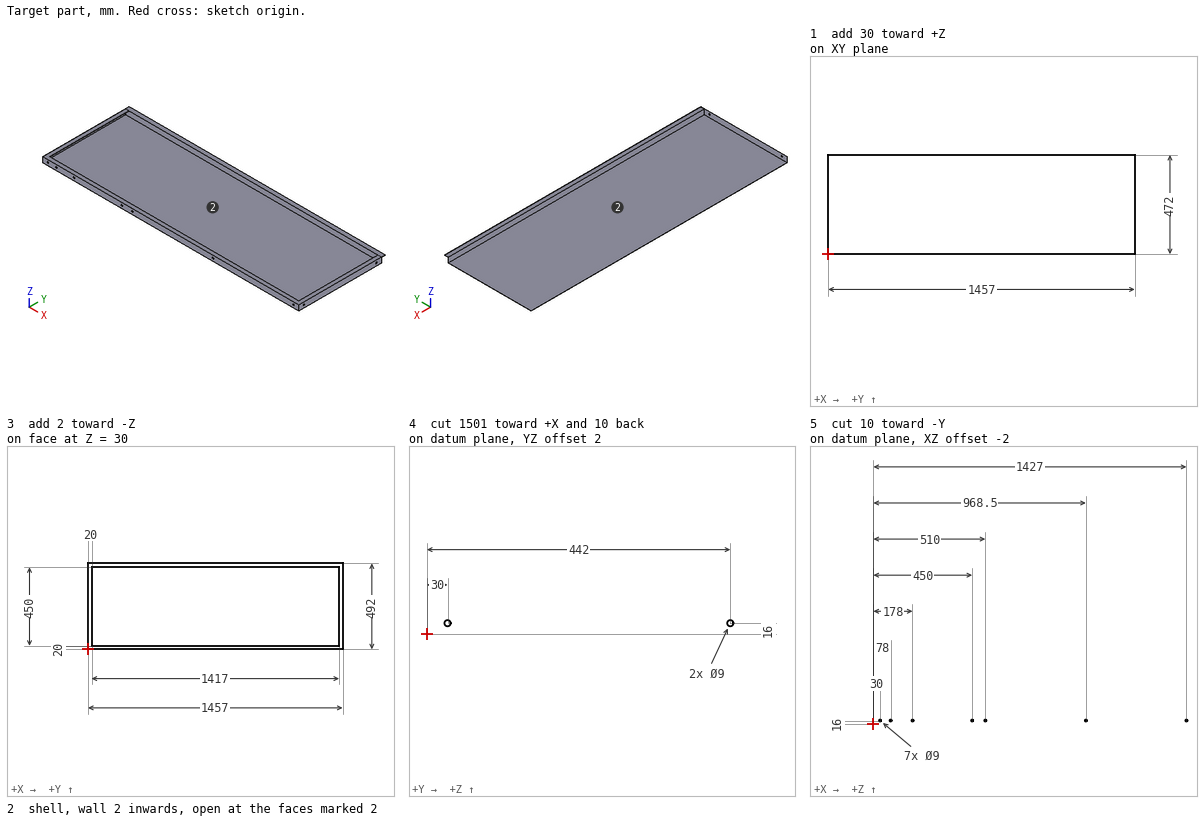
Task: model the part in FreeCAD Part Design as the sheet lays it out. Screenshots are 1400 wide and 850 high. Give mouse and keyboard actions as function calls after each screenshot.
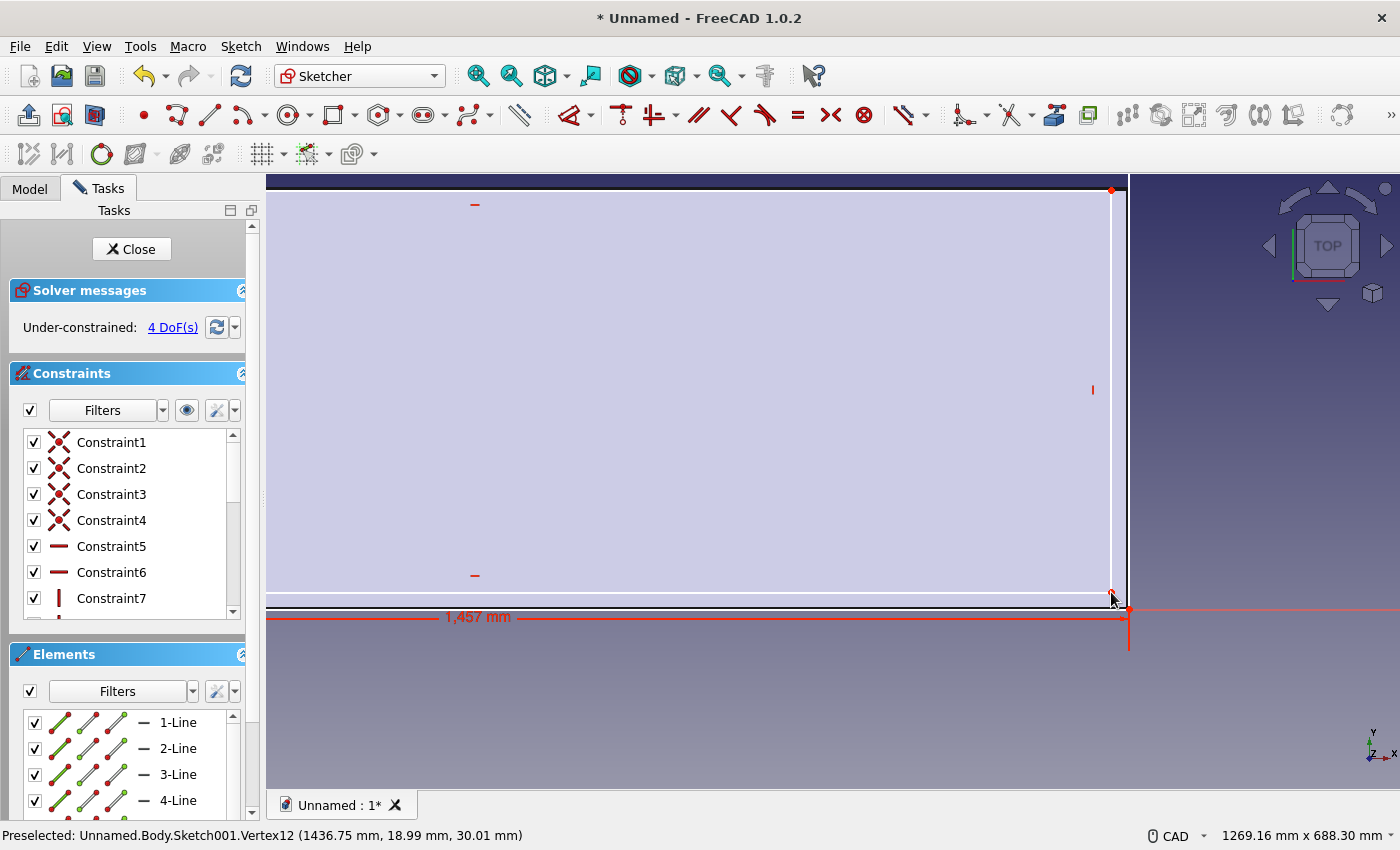
scroll(1113, 593, down, 3)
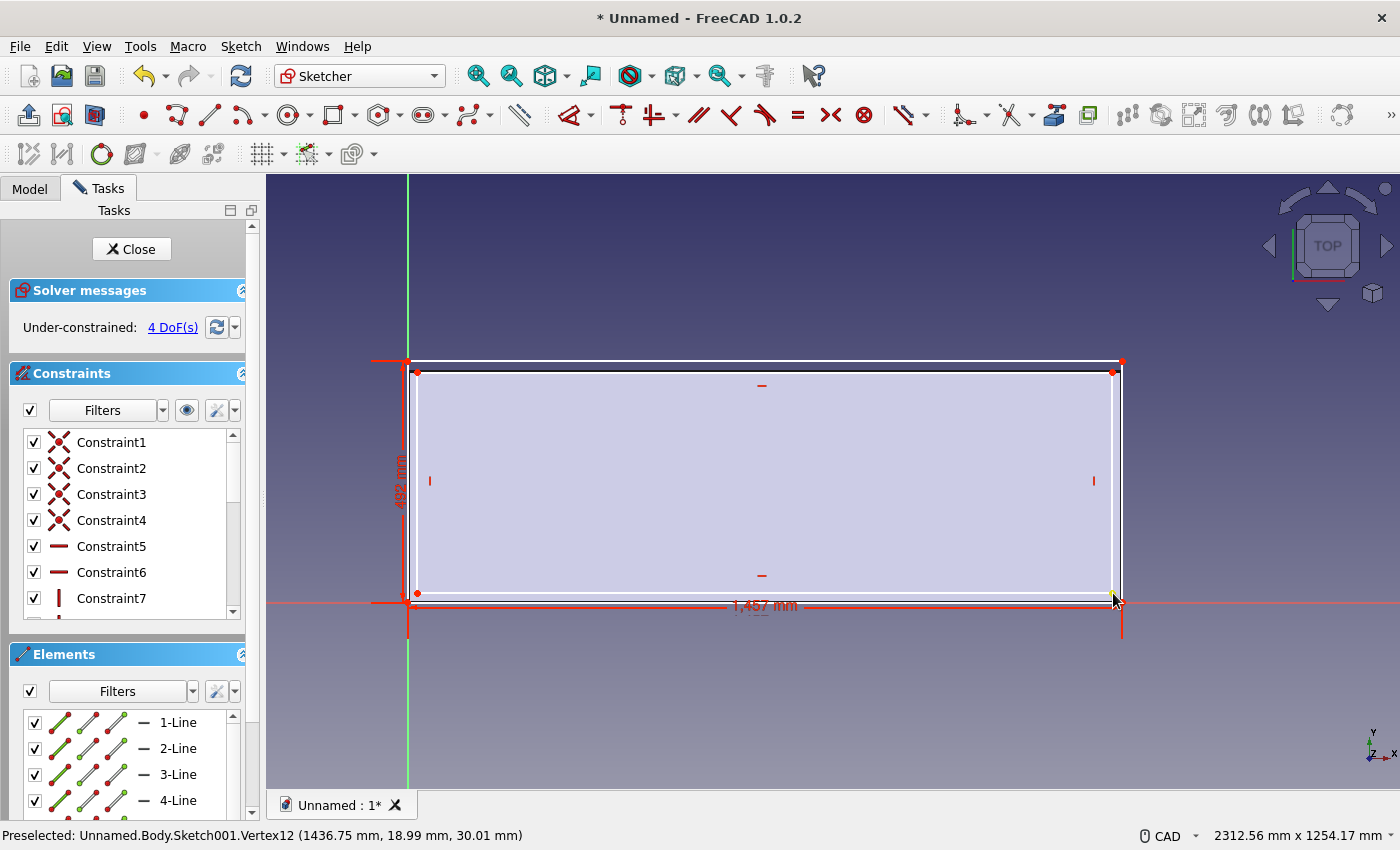
scroll(417, 439, up, 2)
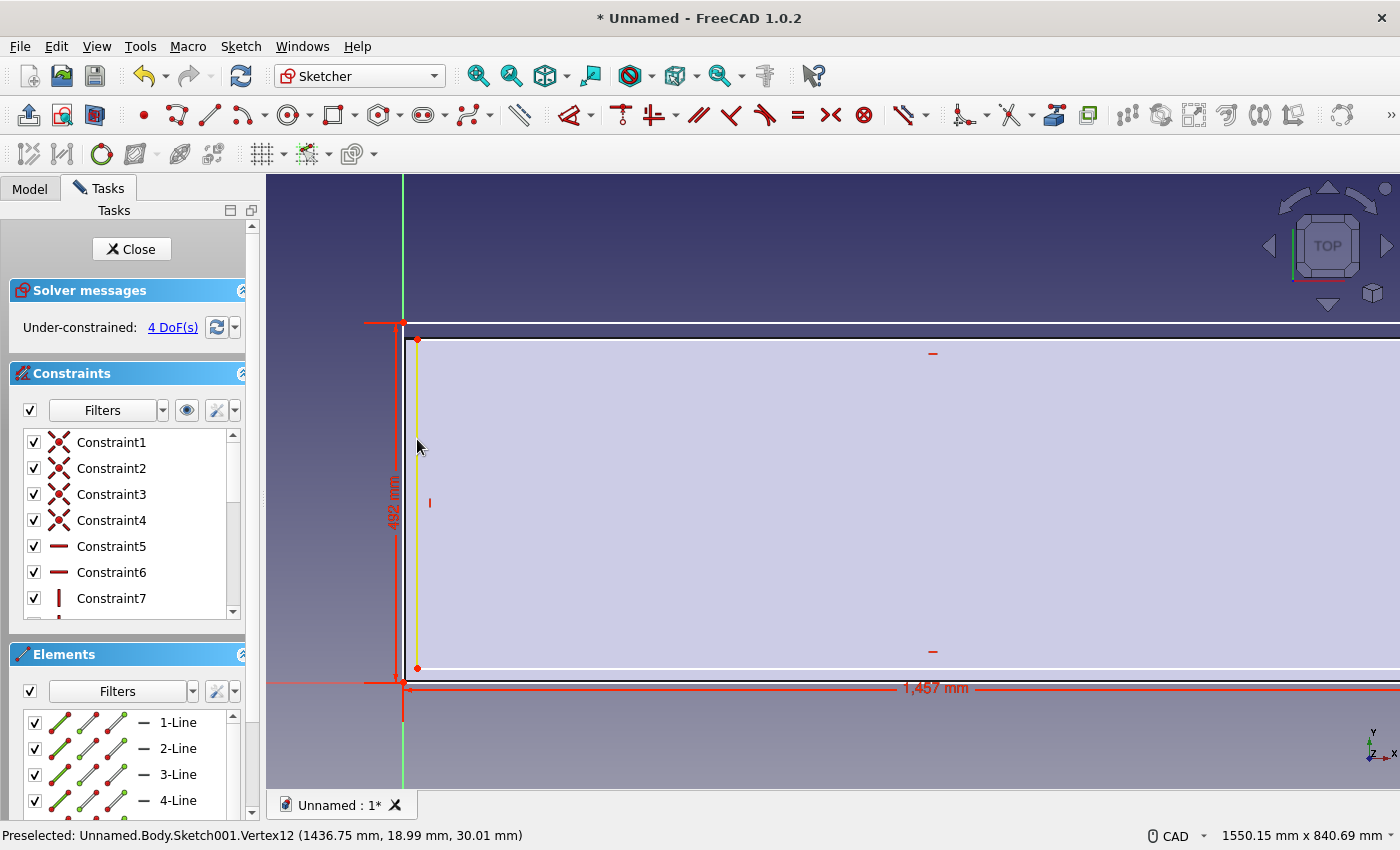
click(417, 438)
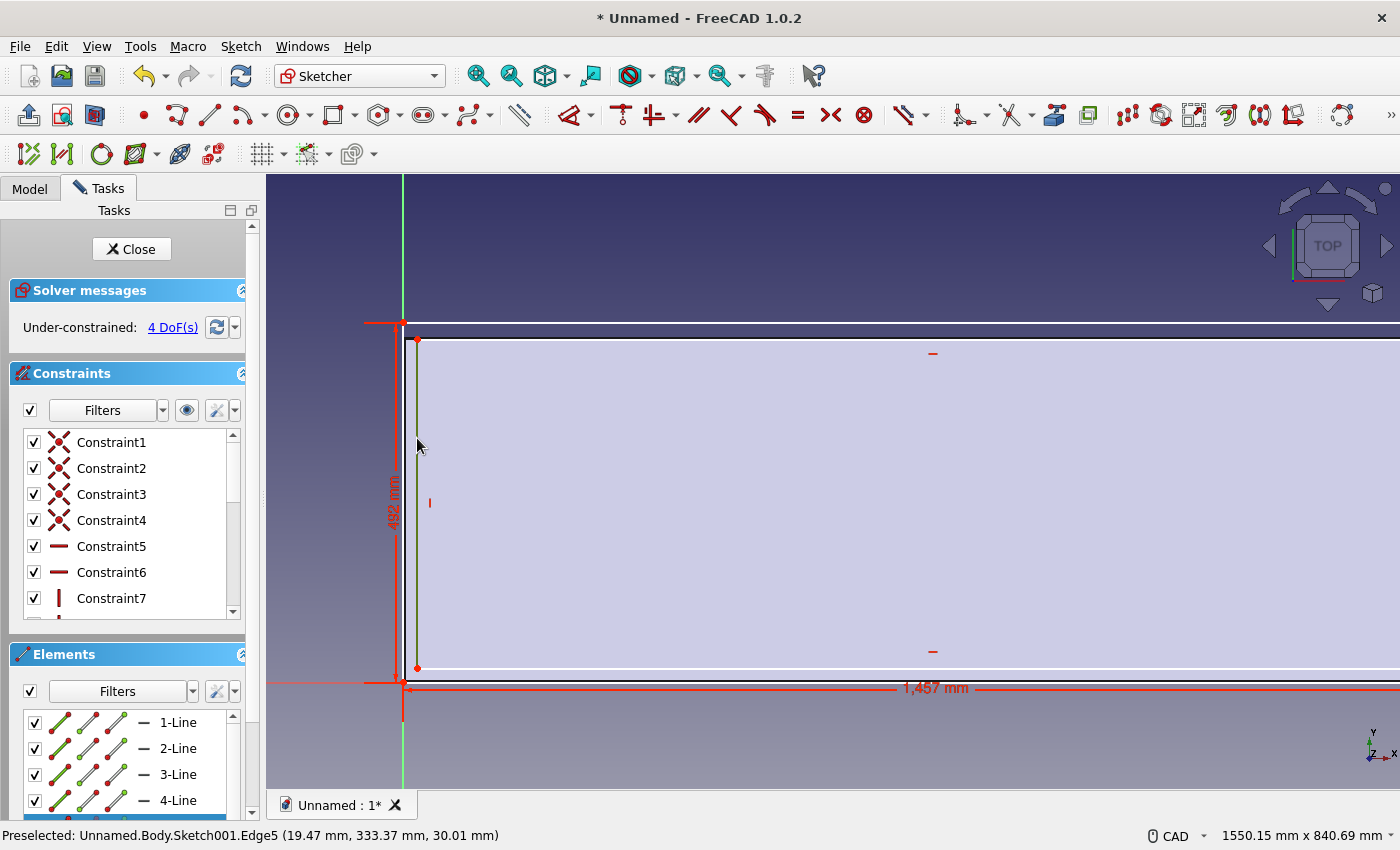
key(i)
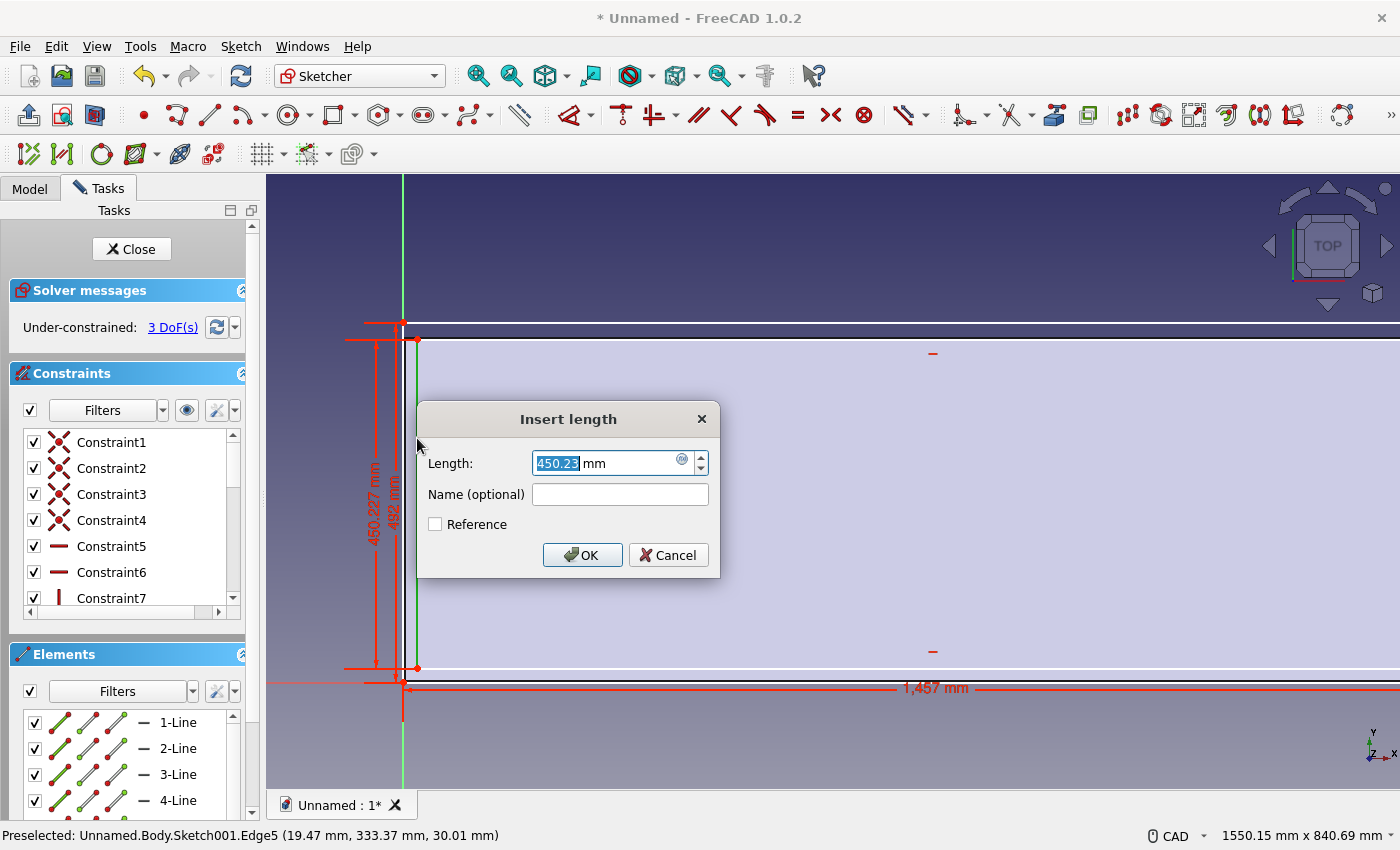
text(450)
key(Return)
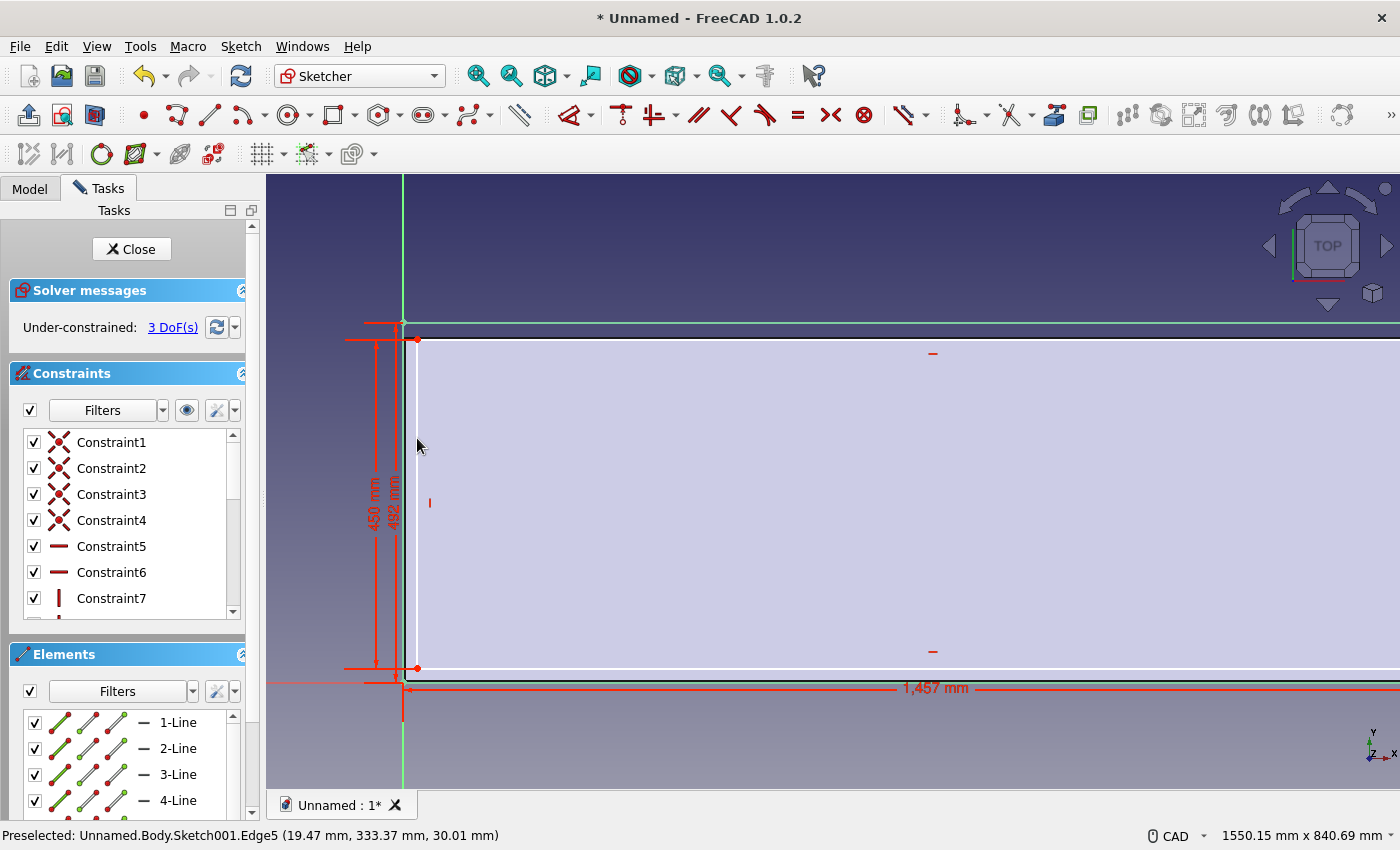
scroll(417, 340, up, 5)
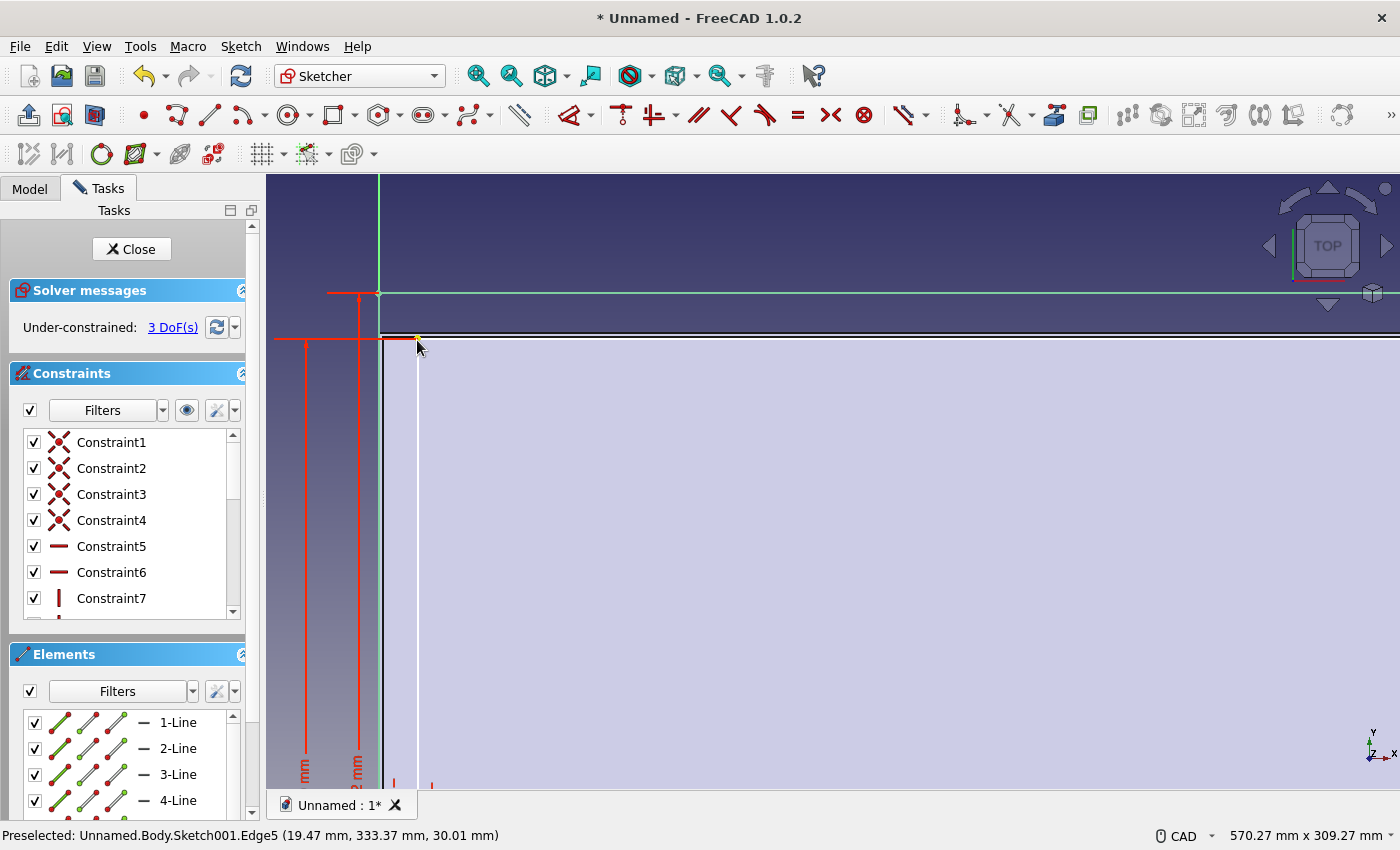
click(418, 339)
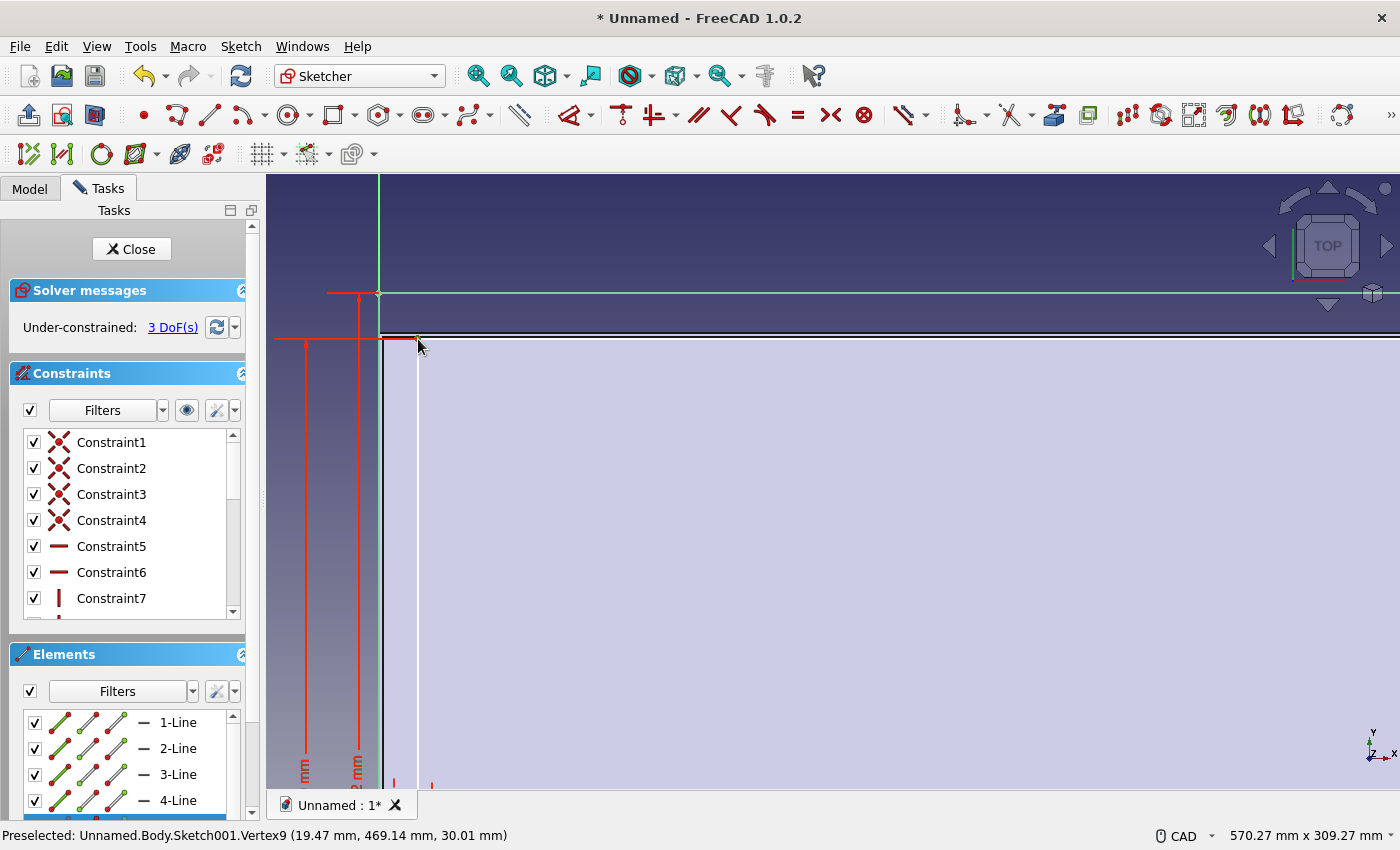
key(l)